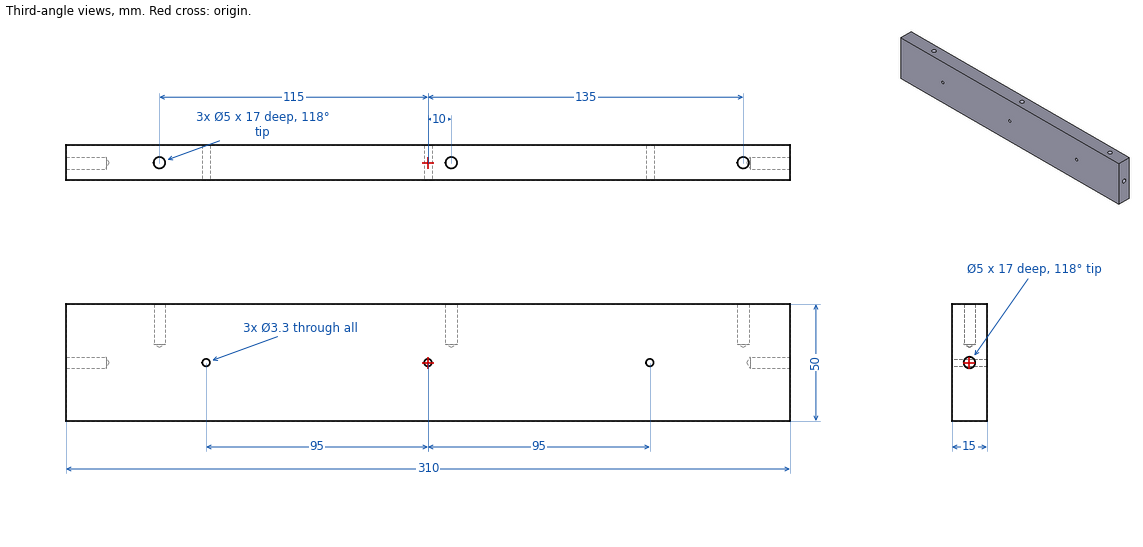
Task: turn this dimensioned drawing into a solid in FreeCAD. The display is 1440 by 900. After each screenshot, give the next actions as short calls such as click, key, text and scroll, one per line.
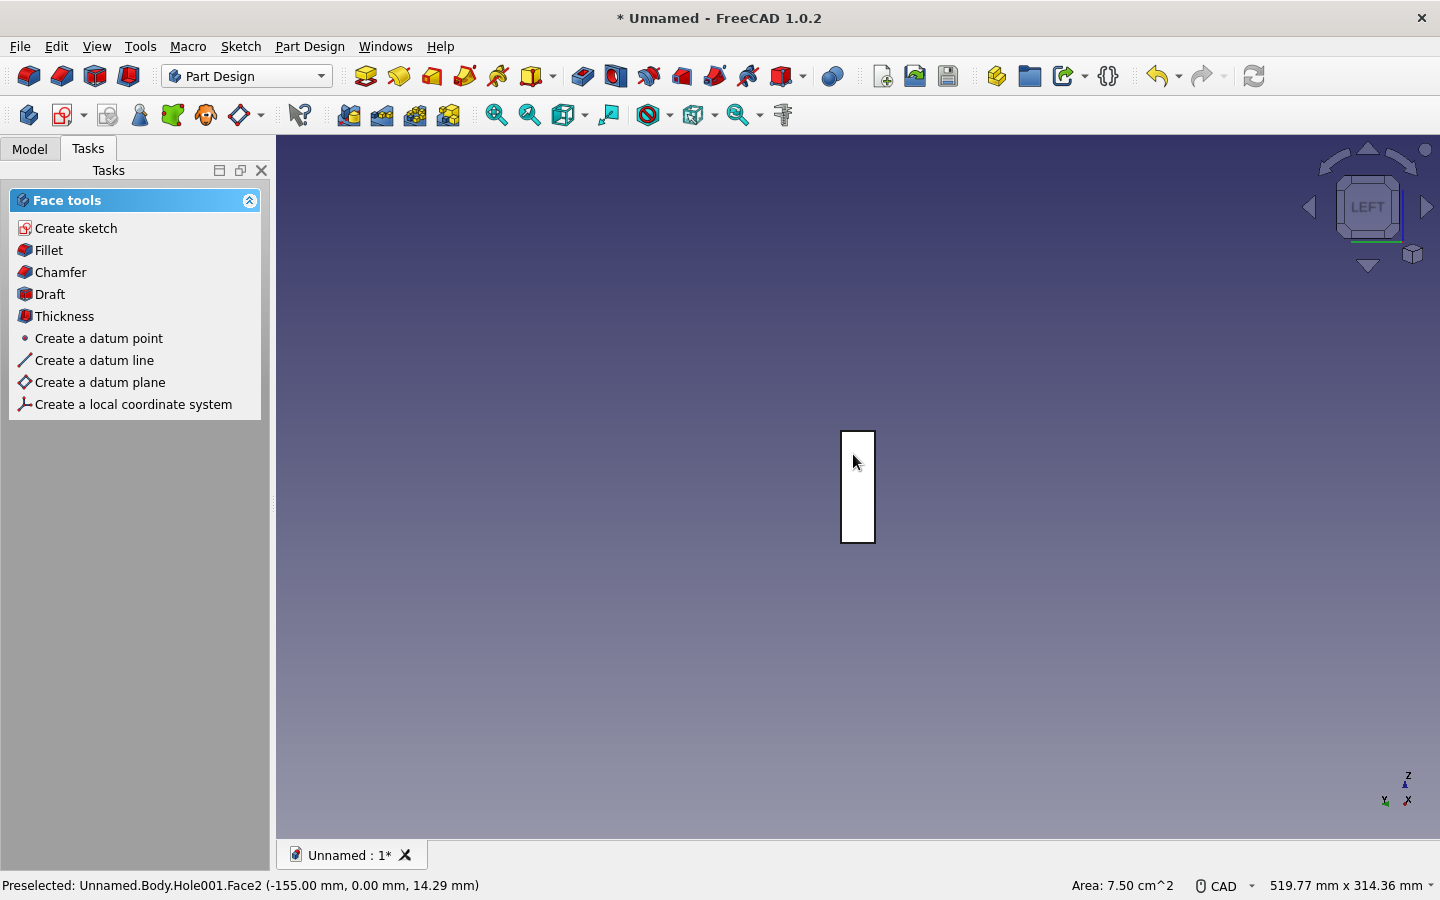
click(62, 116)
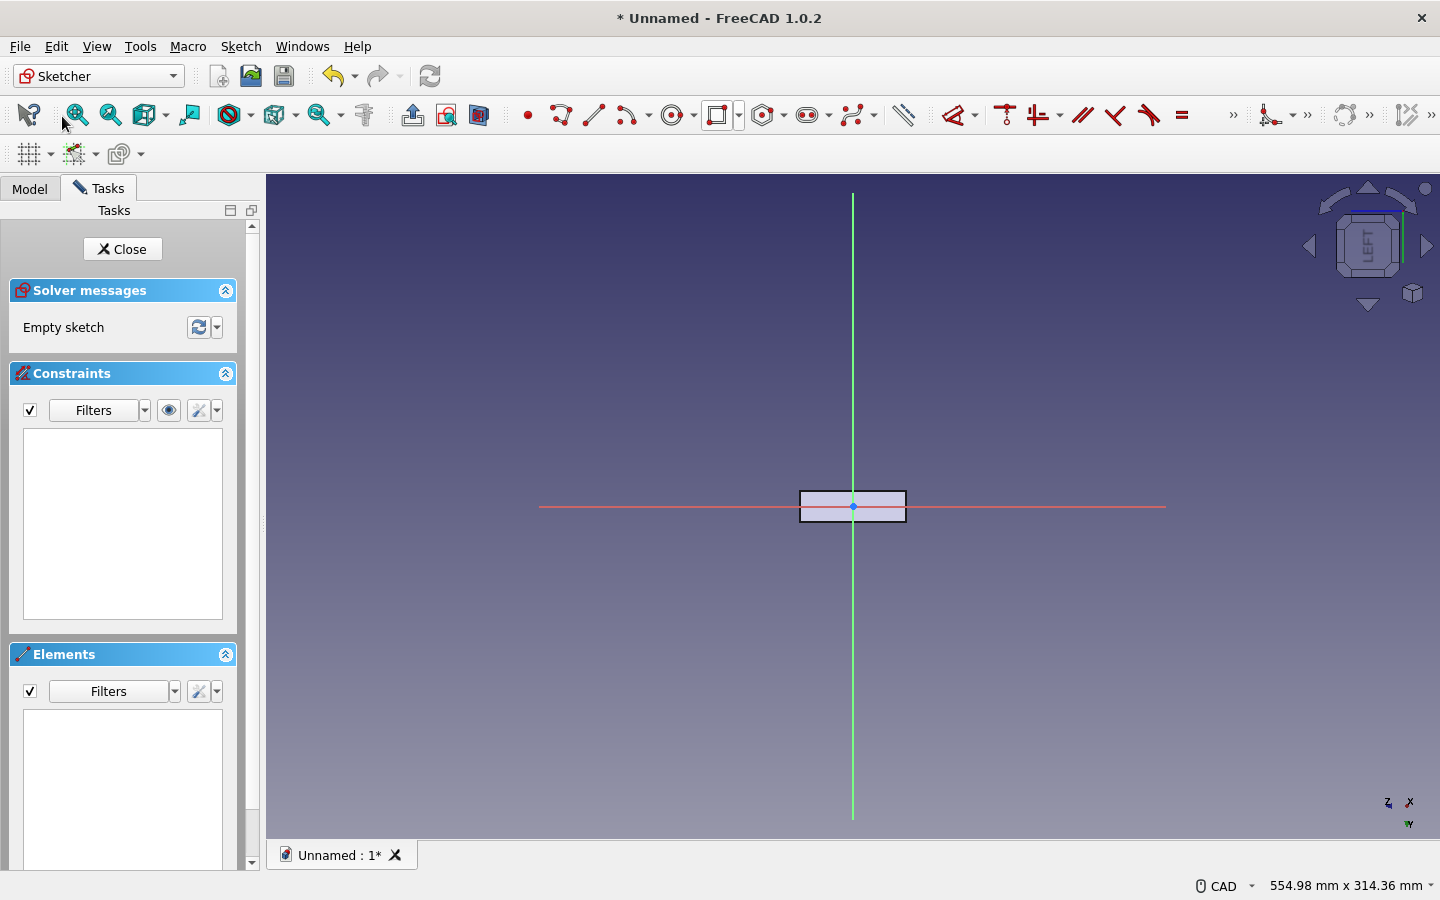
scroll(857, 506, up, 15)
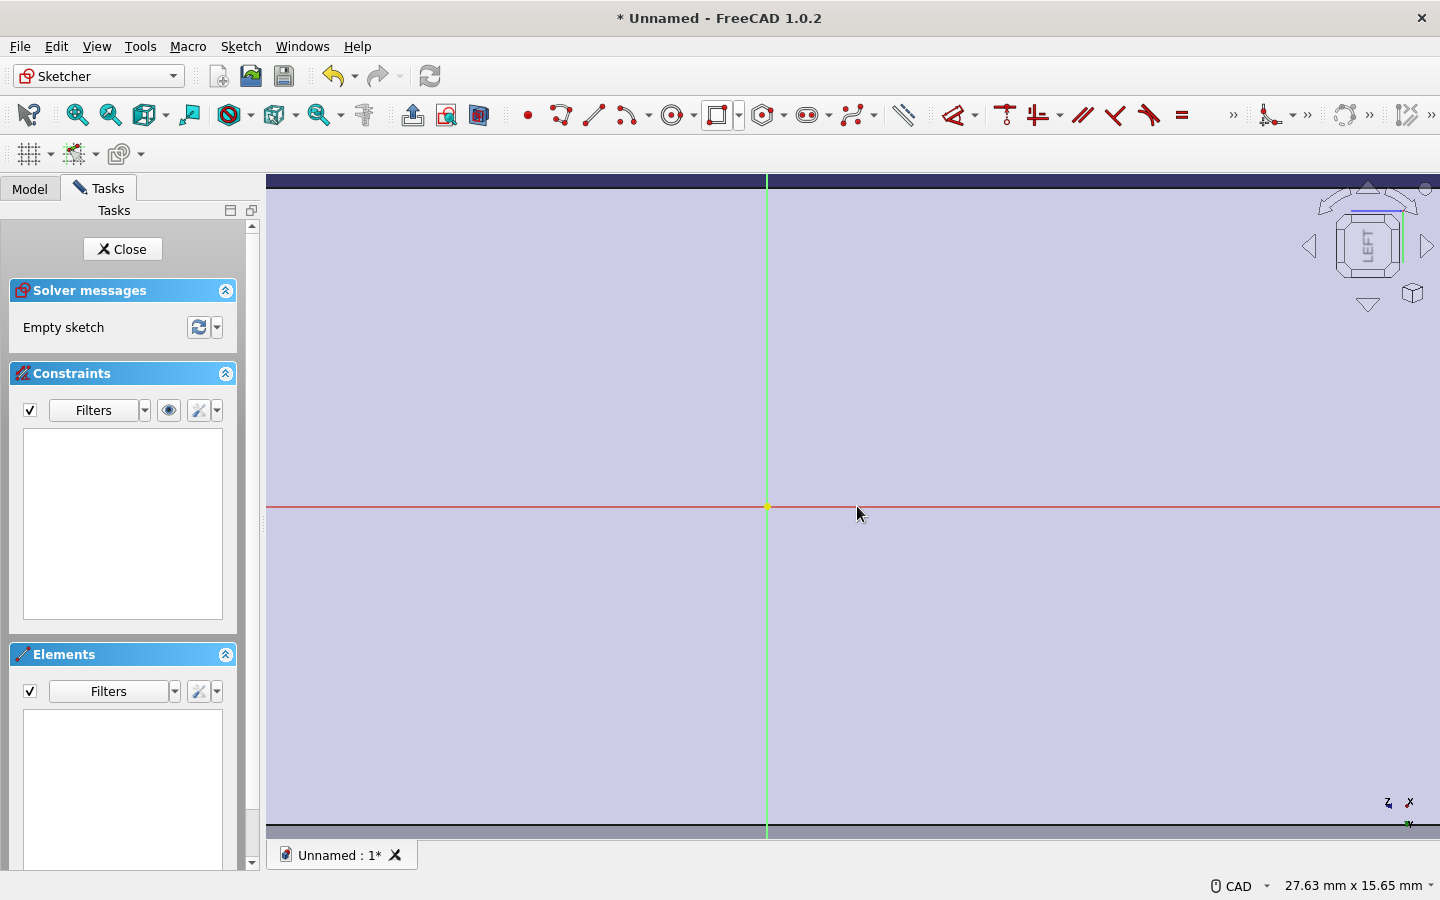
scroll(753, 506, up, 4)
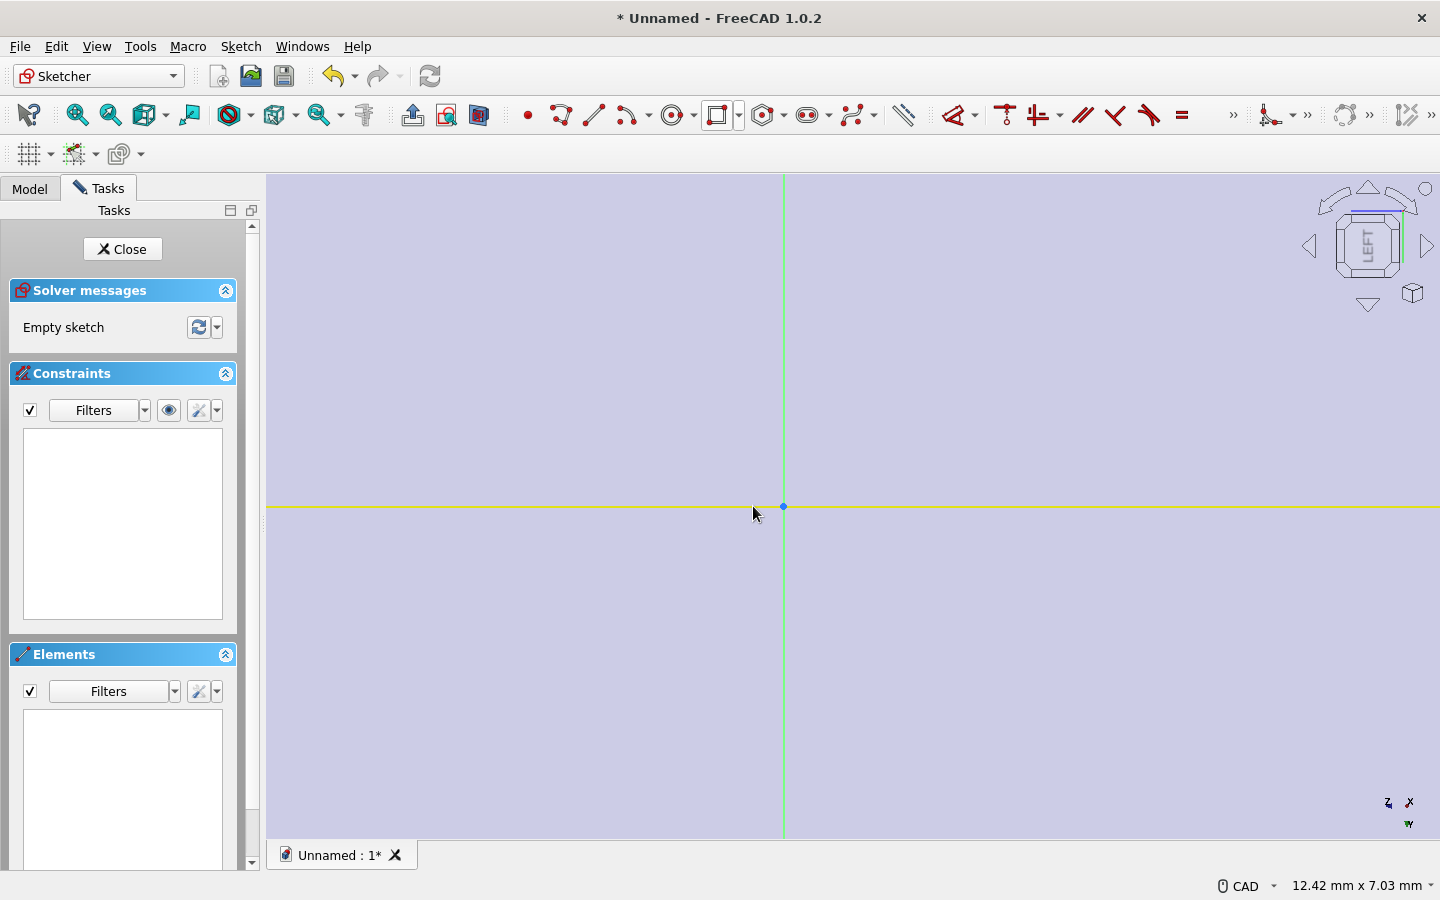
click(672, 116)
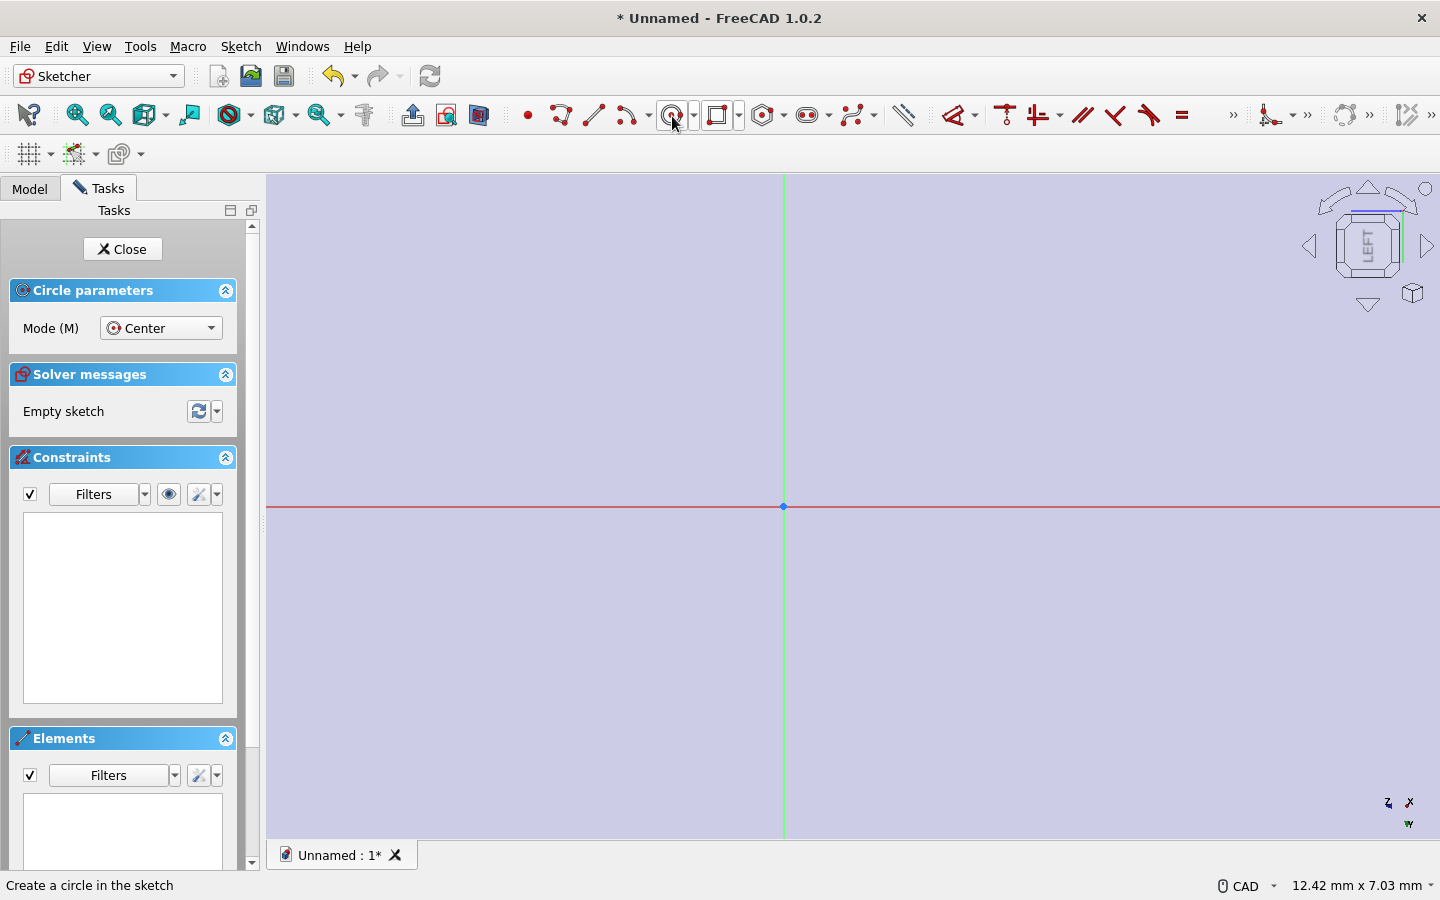
click(784, 506)
click(951, 339)
key(Escape)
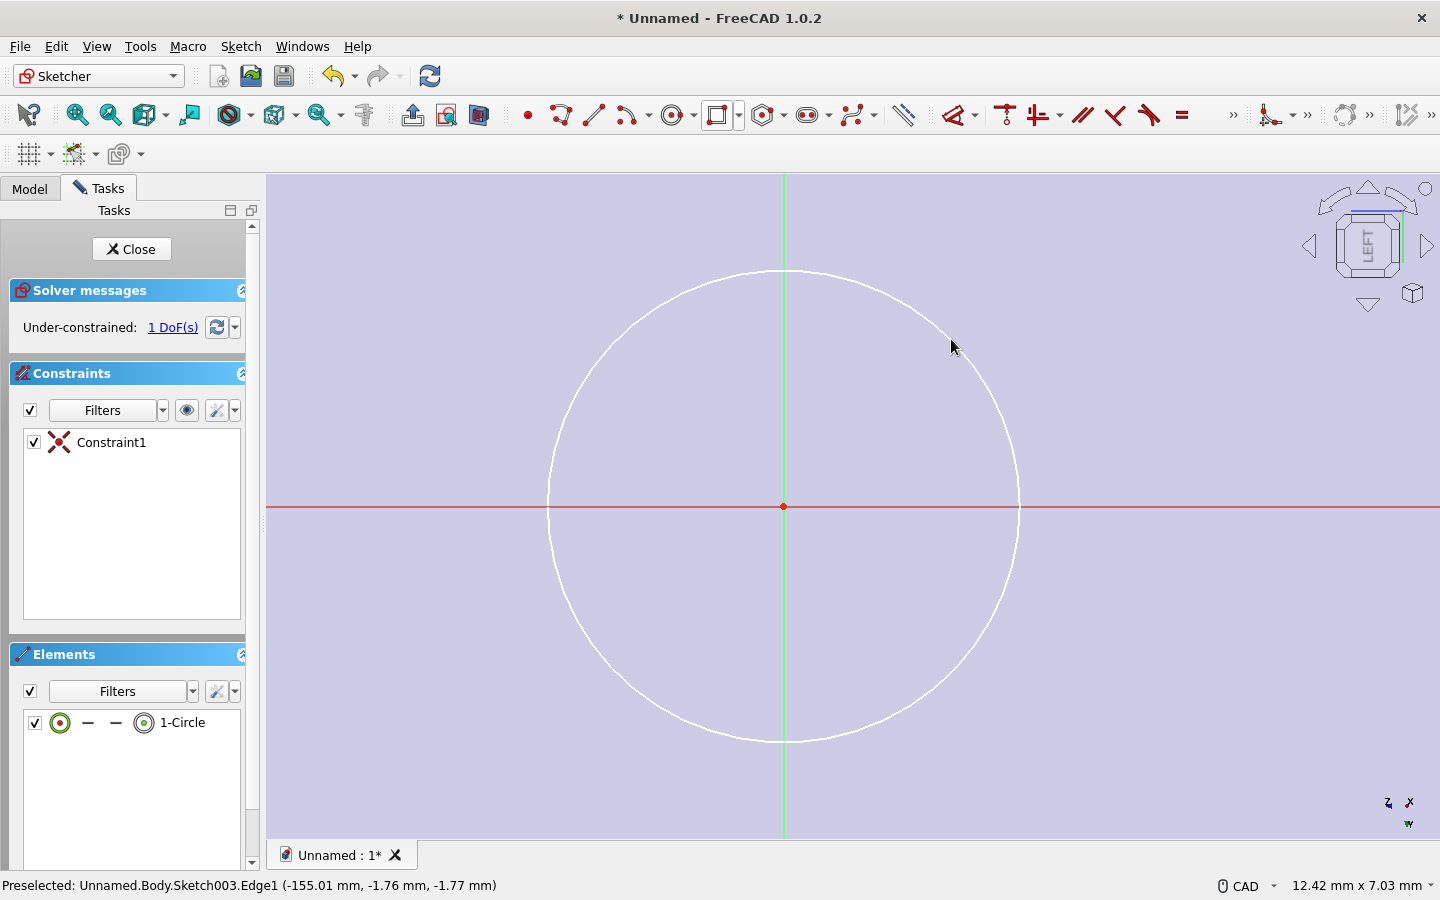
click(952, 116)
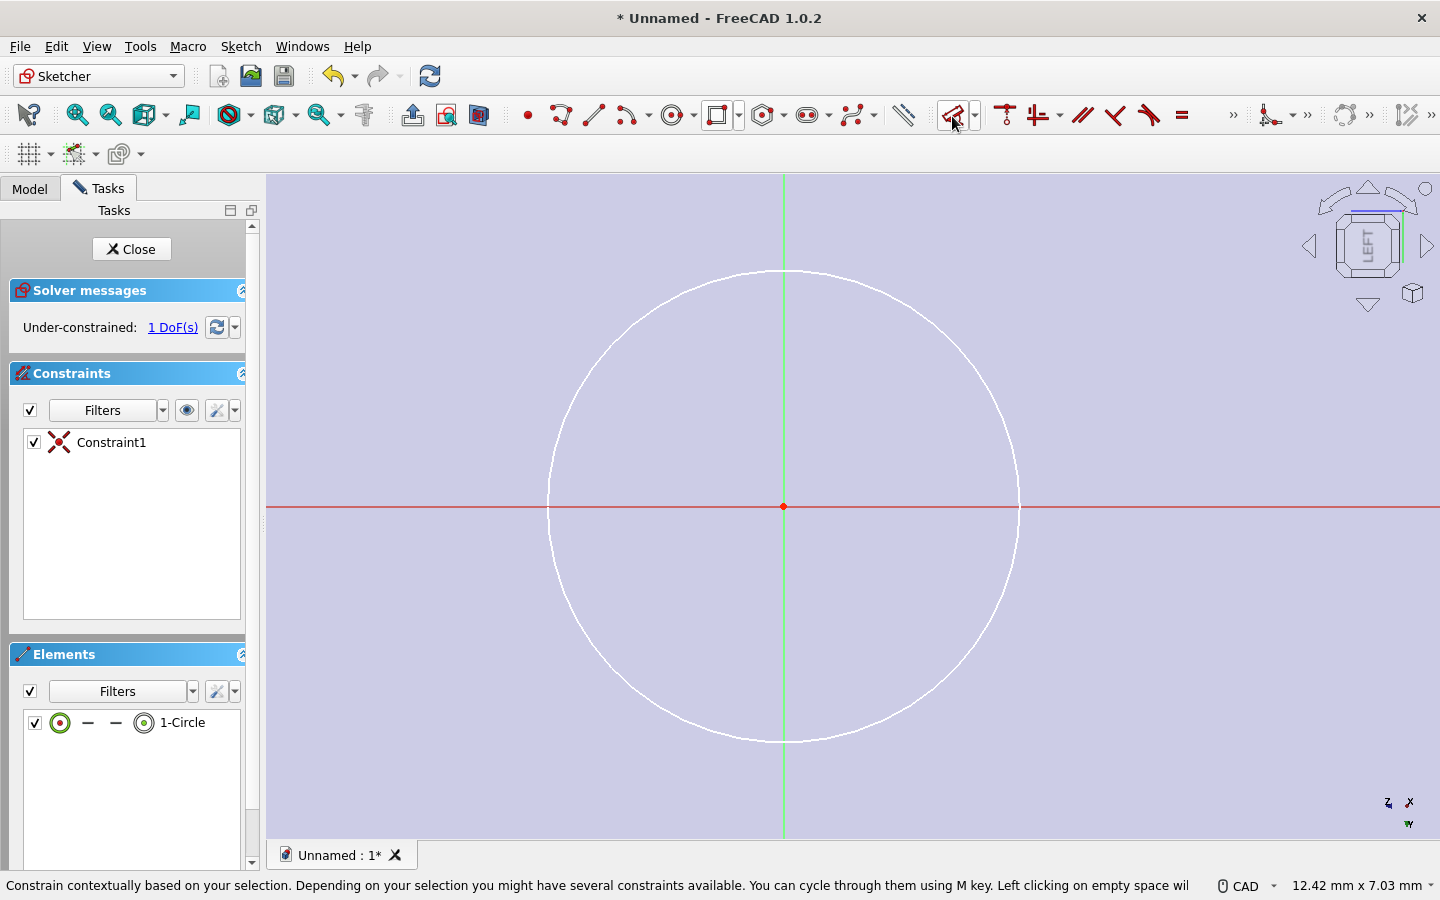
click(950, 339)
click(973, 316)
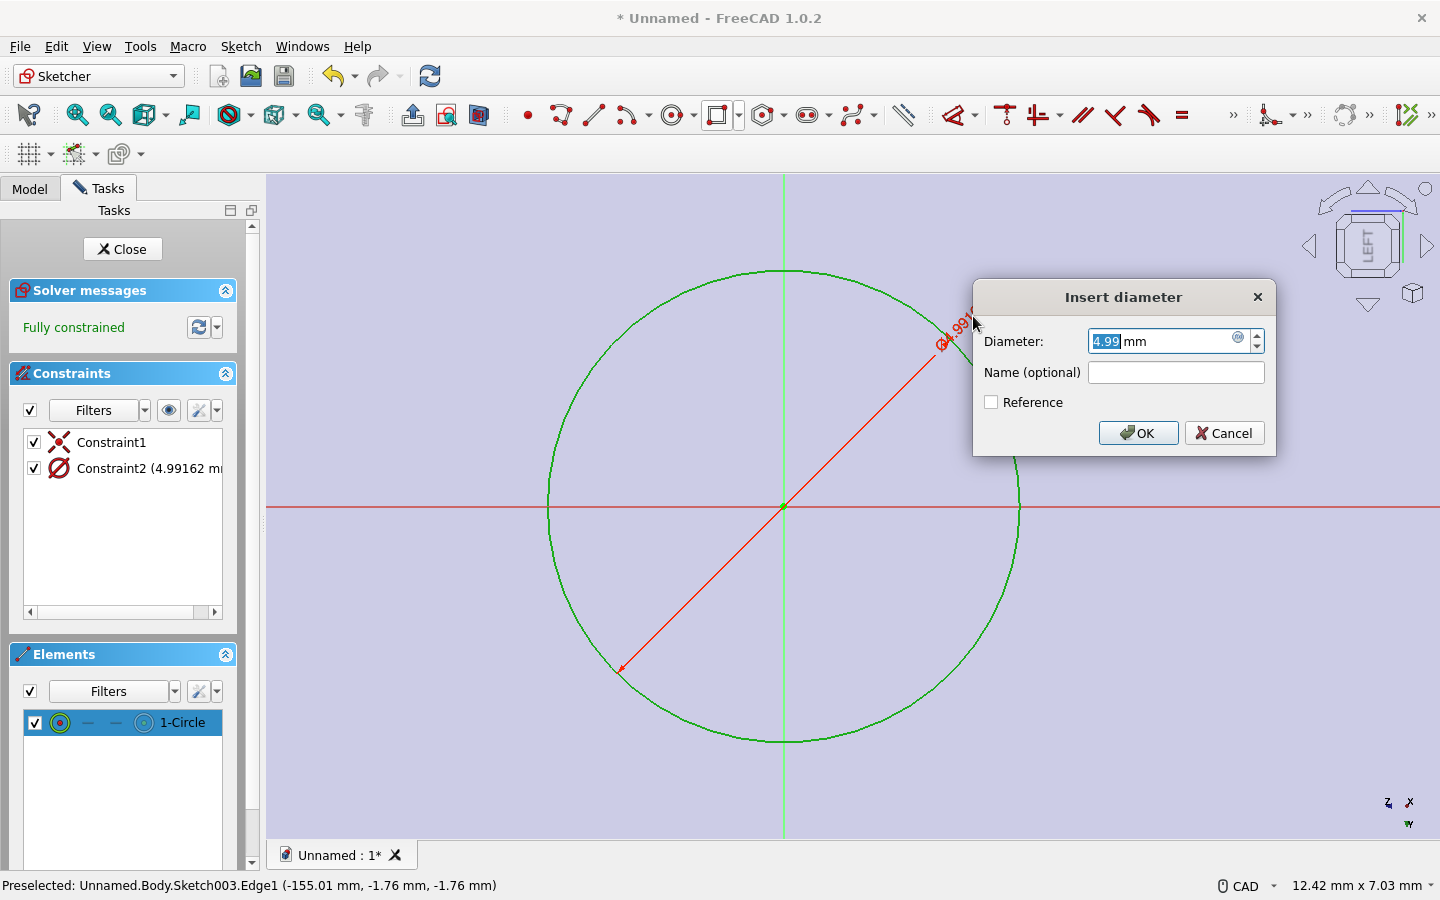
text(5)
key(Return)
key(Escape)